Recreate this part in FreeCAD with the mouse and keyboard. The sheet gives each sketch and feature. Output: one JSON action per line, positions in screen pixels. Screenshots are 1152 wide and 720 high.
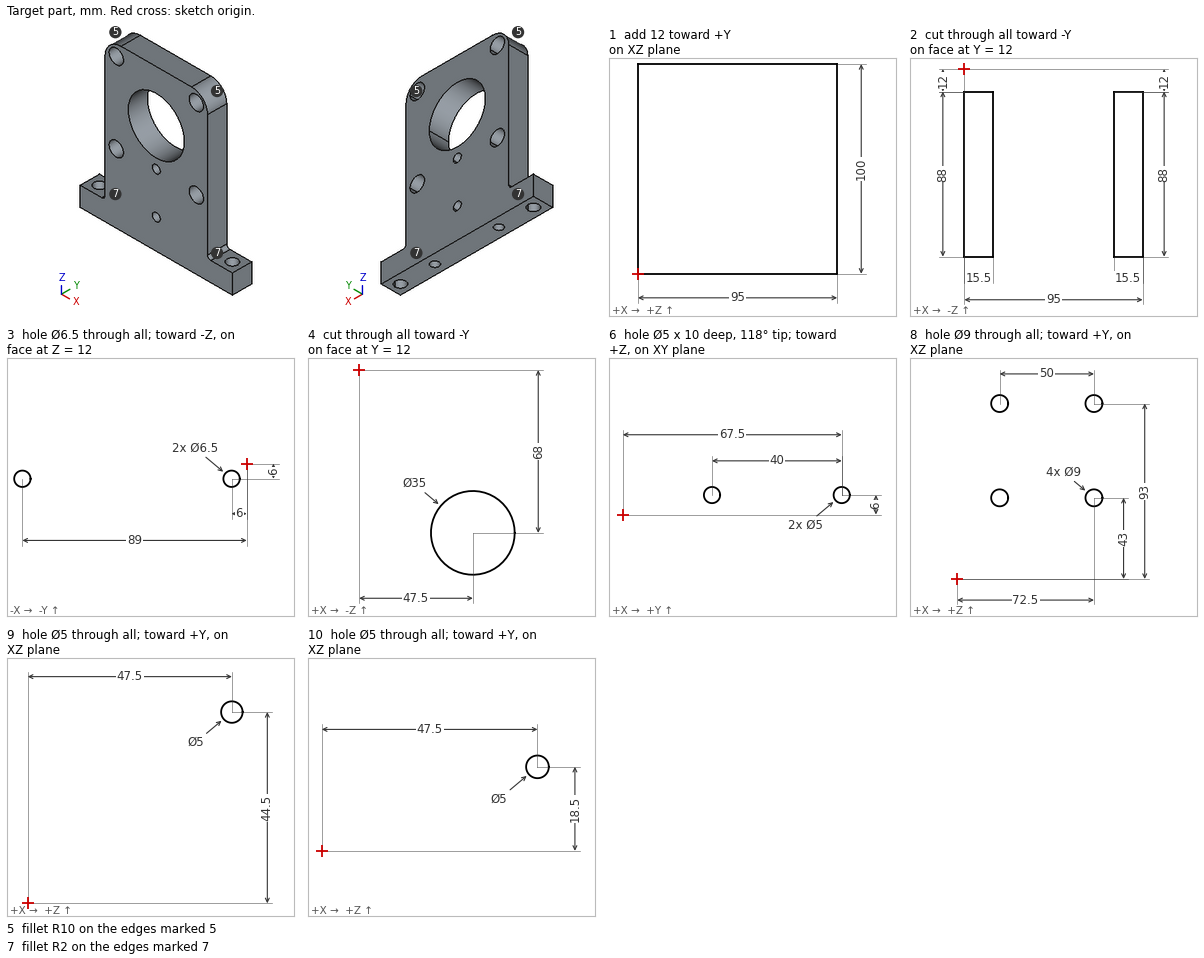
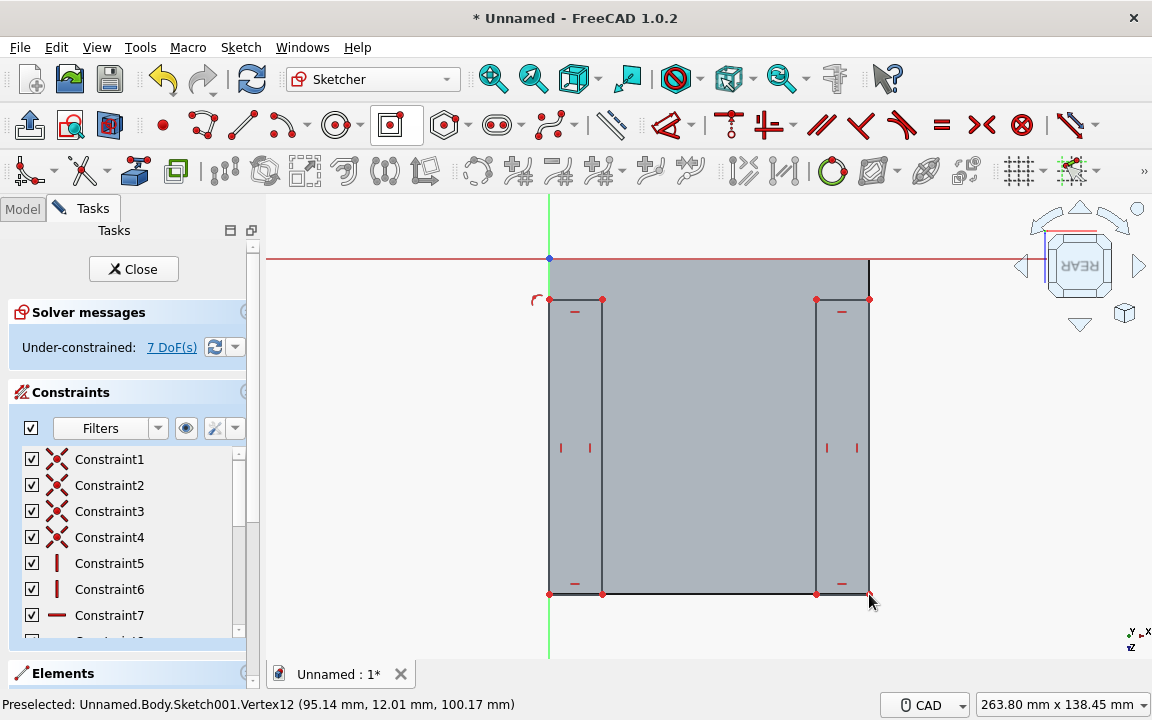
{"action": "left_click", "coordinate": [666, 126]}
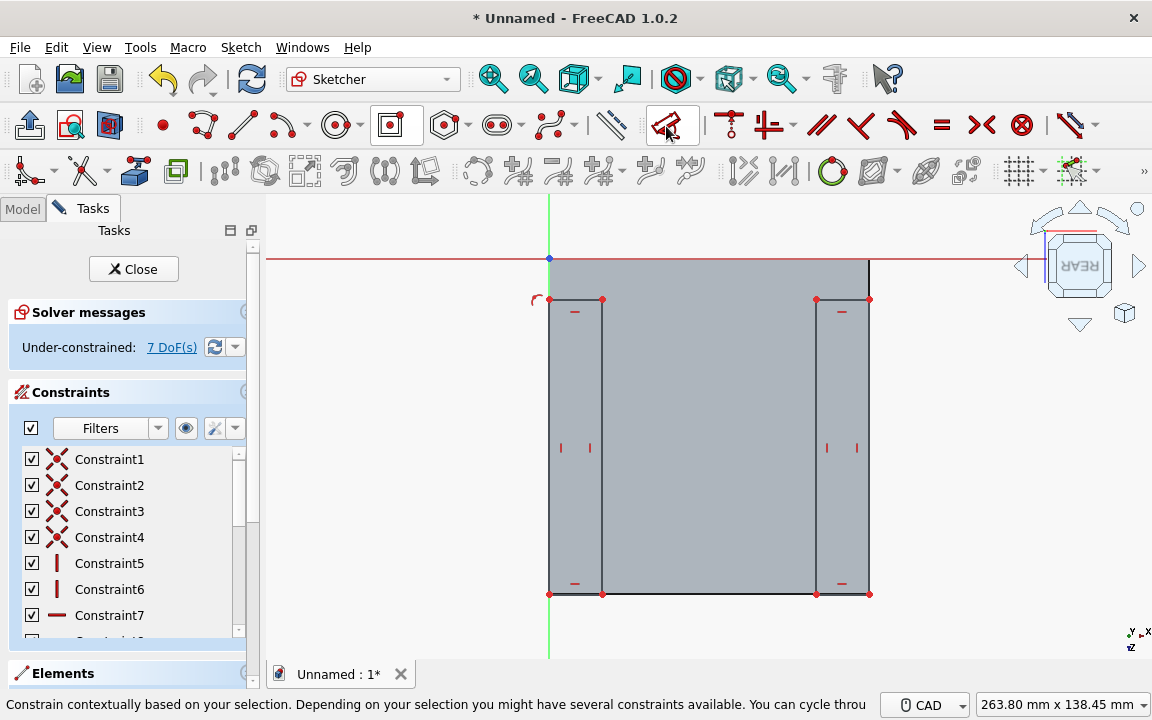
{"action": "left_click", "coordinate": [549, 389]}
{"action": "left_click", "coordinate": [515, 448]}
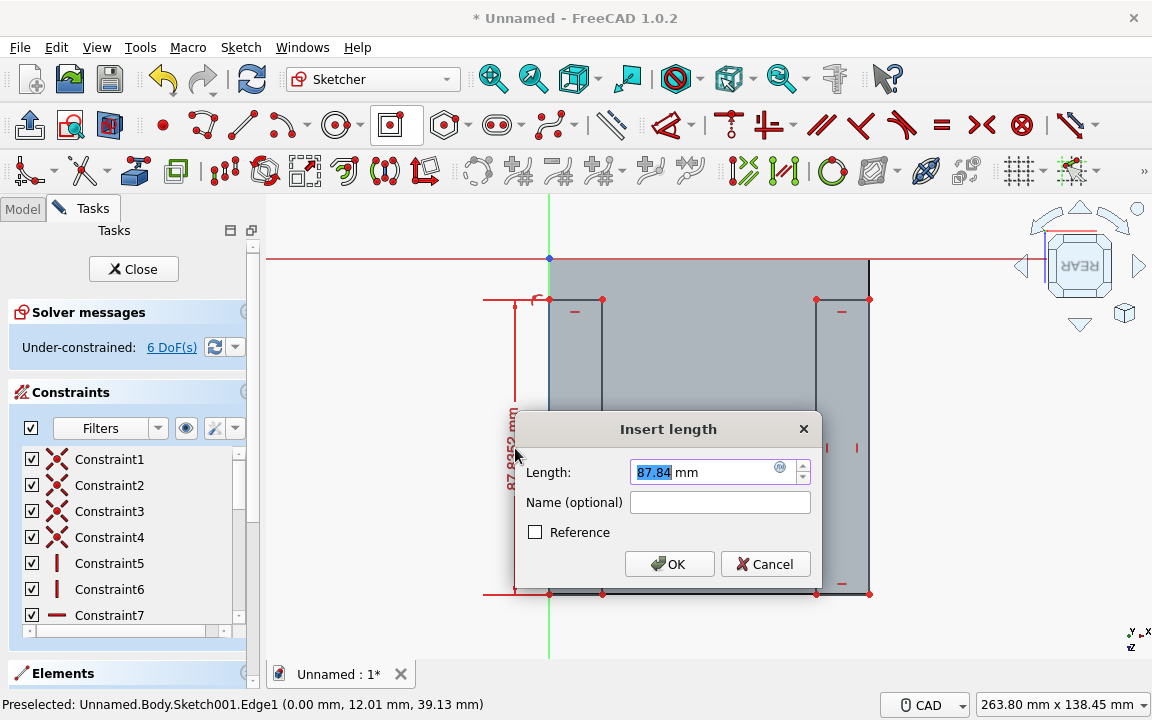
{"action": "type", "text": "88"}
{"action": "key", "text": "Return"}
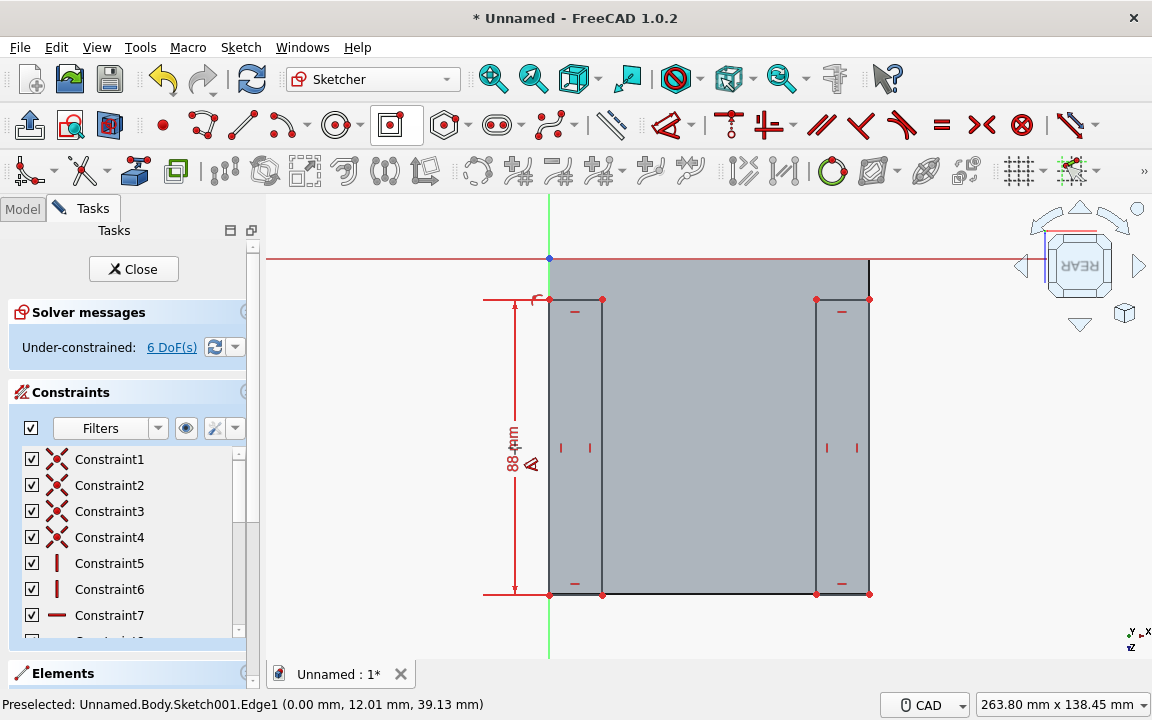
{"action": "left_click", "coordinate": [816, 389]}
{"action": "left_click", "coordinate": [850, 448]}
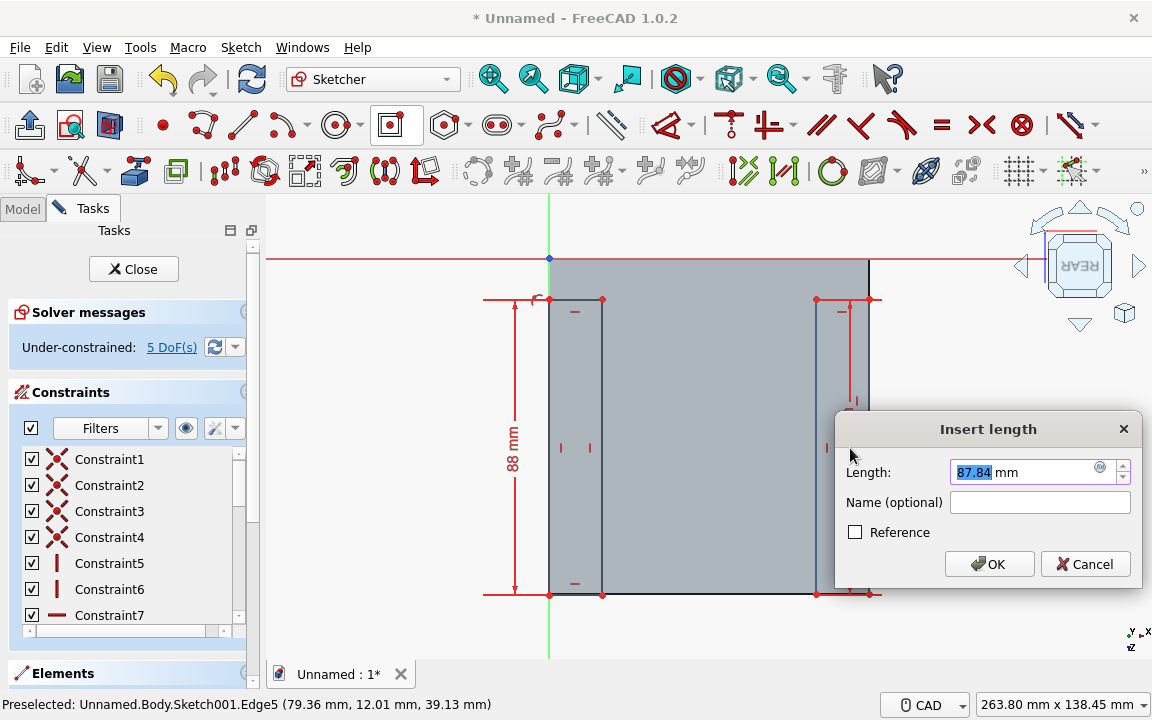
{"action": "type", "text": "88"}
{"action": "key", "text": "Return"}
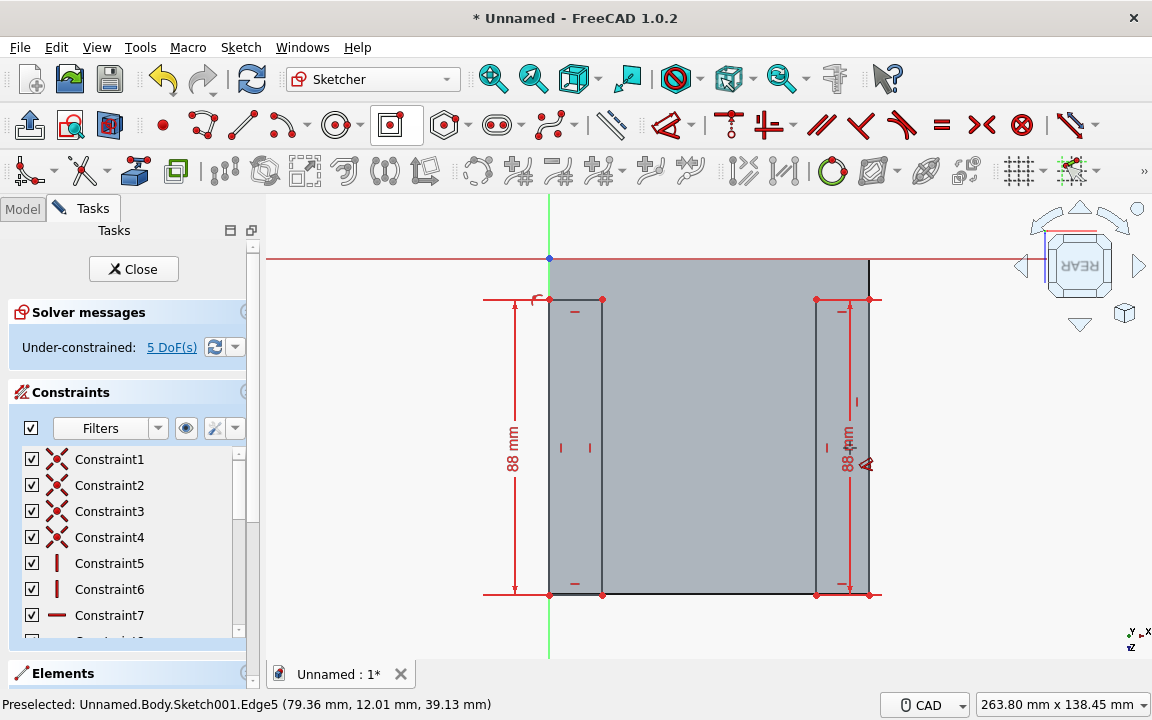
{"action": "left_click", "coordinate": [549, 300]}
{"action": "left_click", "coordinate": [515, 279]}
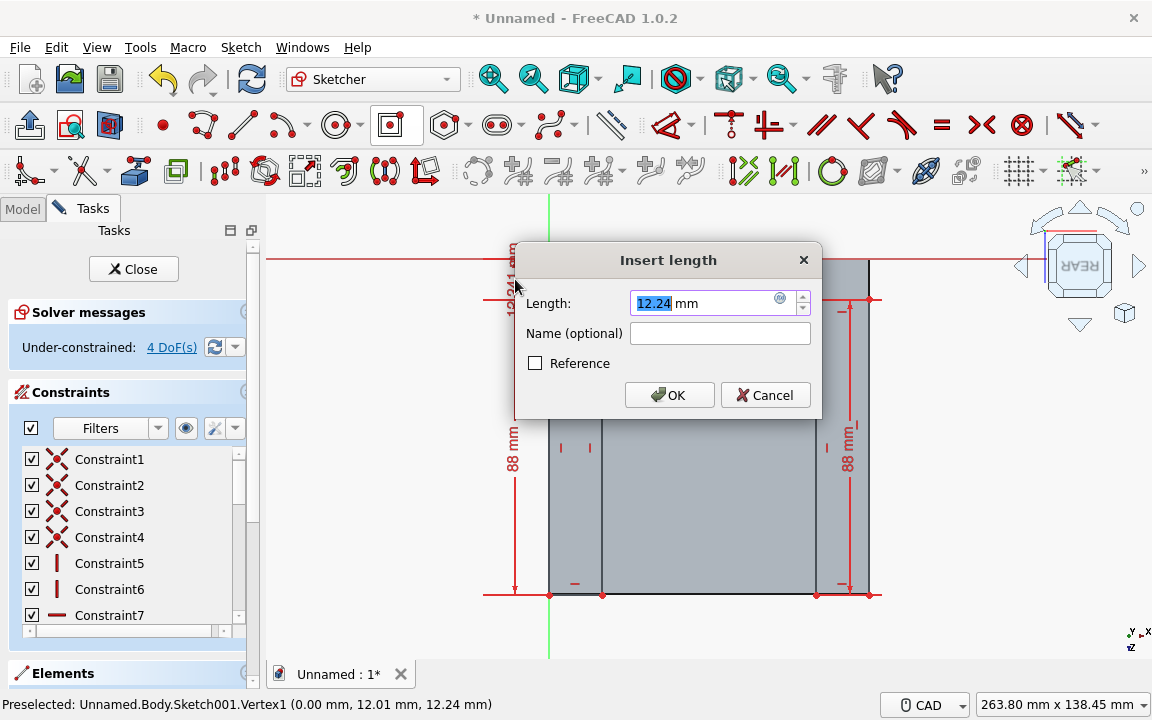
{"action": "type", "text": "12"}
{"action": "key", "text": "Return"}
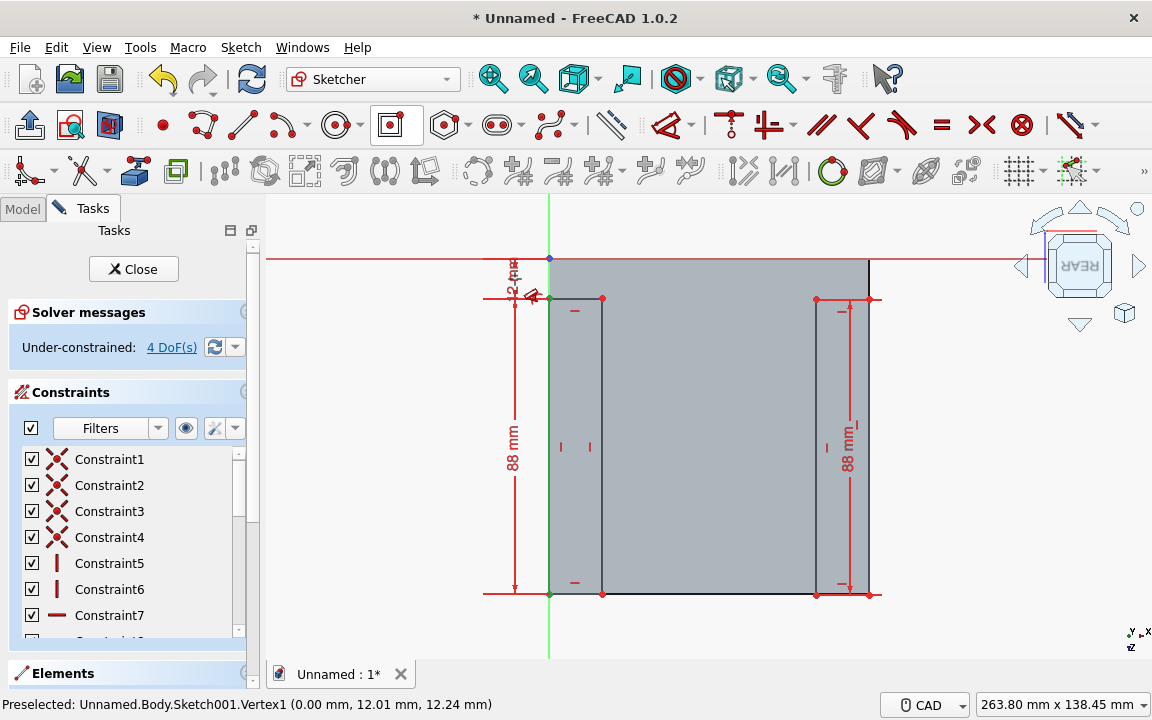
{"action": "left_click", "coordinate": [816, 300]}
{"action": "left_click", "coordinate": [850, 279]}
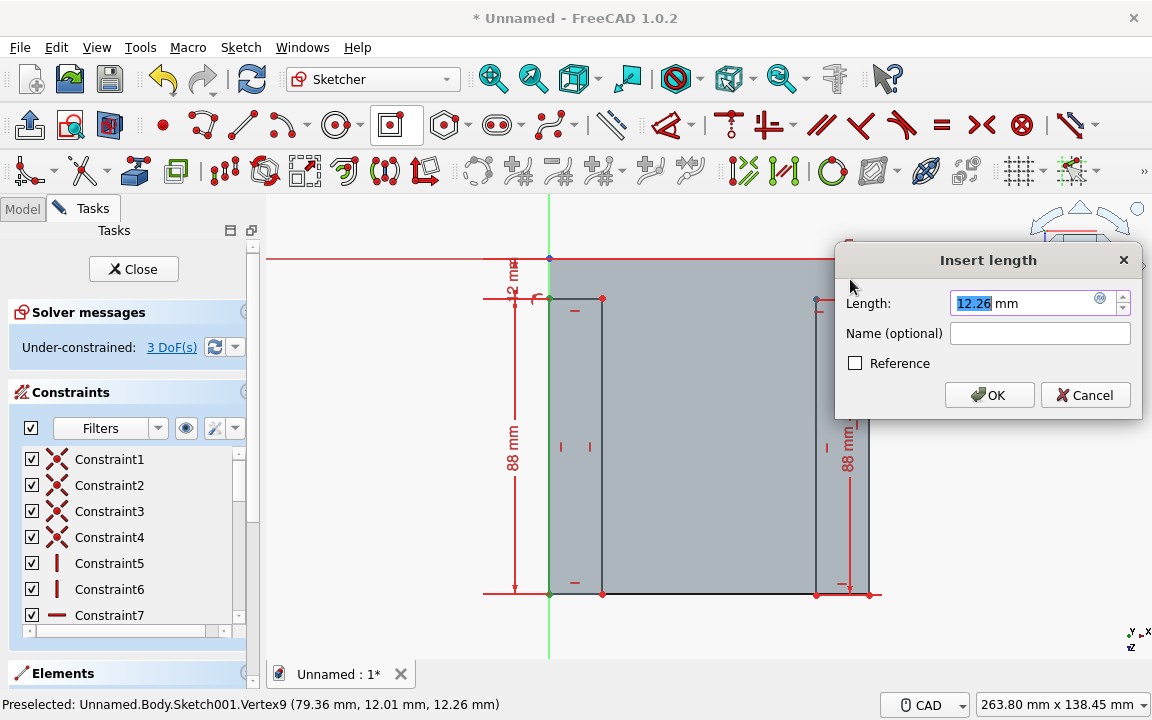
{"action": "type", "text": "12"}
{"action": "key", "text": "Return"}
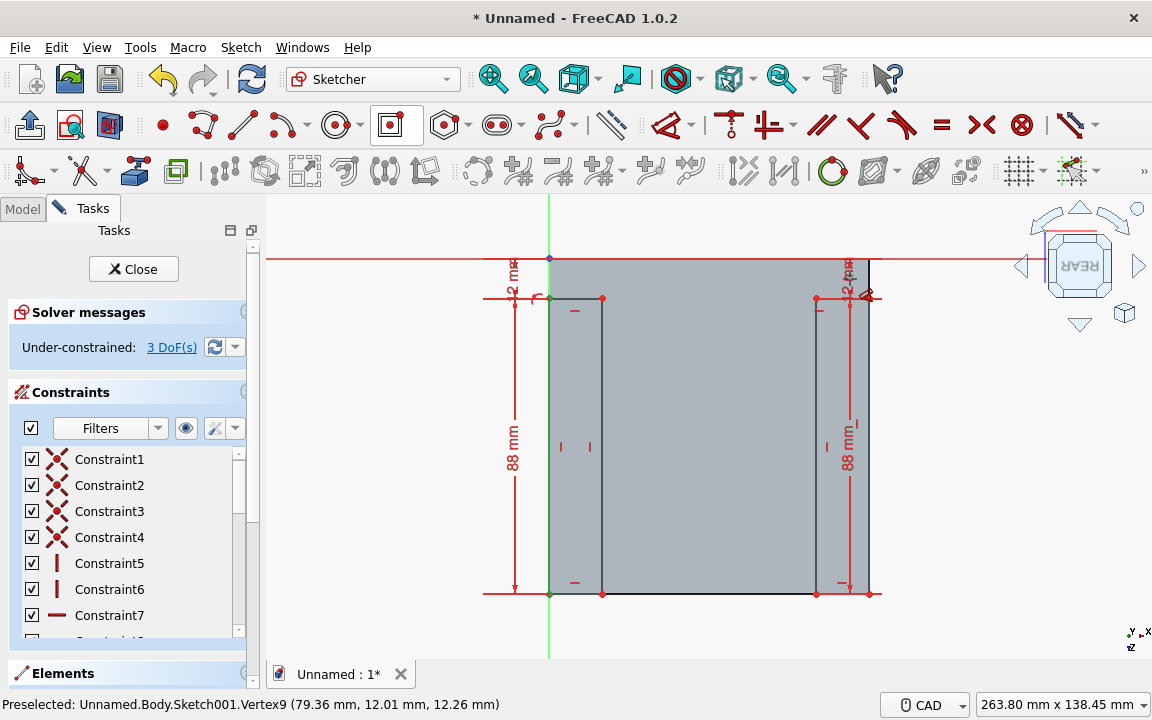
{"action": "left_click", "coordinate": [869, 594]}
{"action": "left_click", "coordinate": [709, 628]}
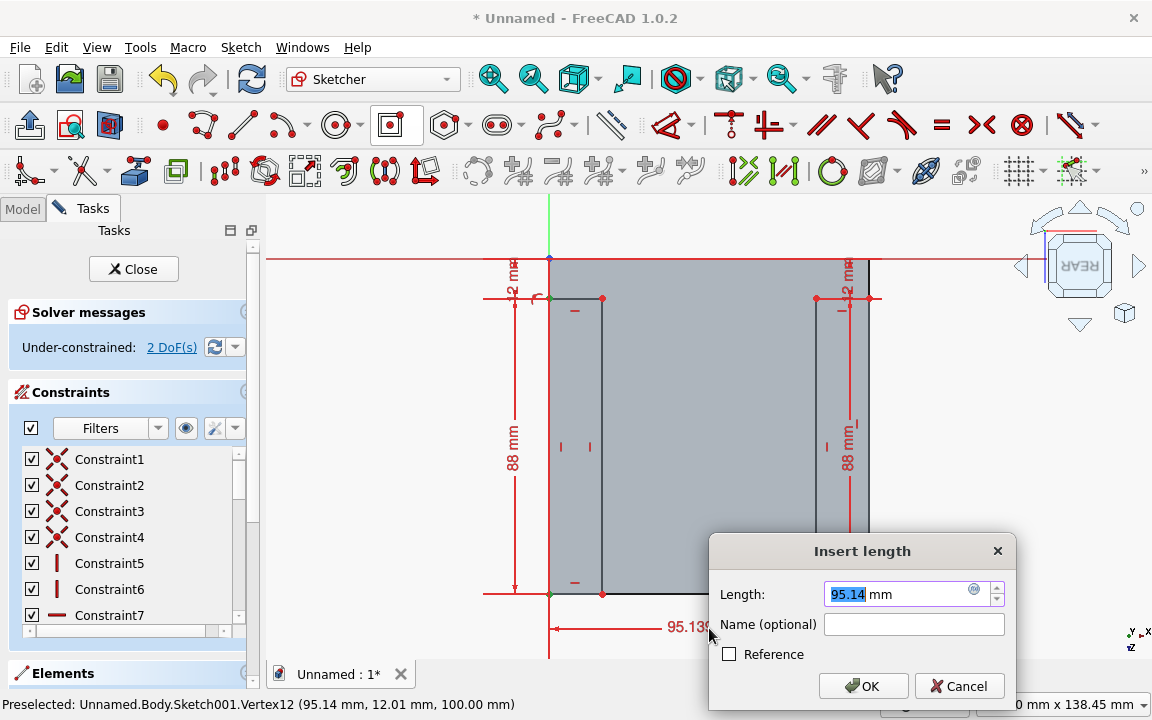
{"action": "type", "text": "95"}
{"action": "key", "text": "Return"}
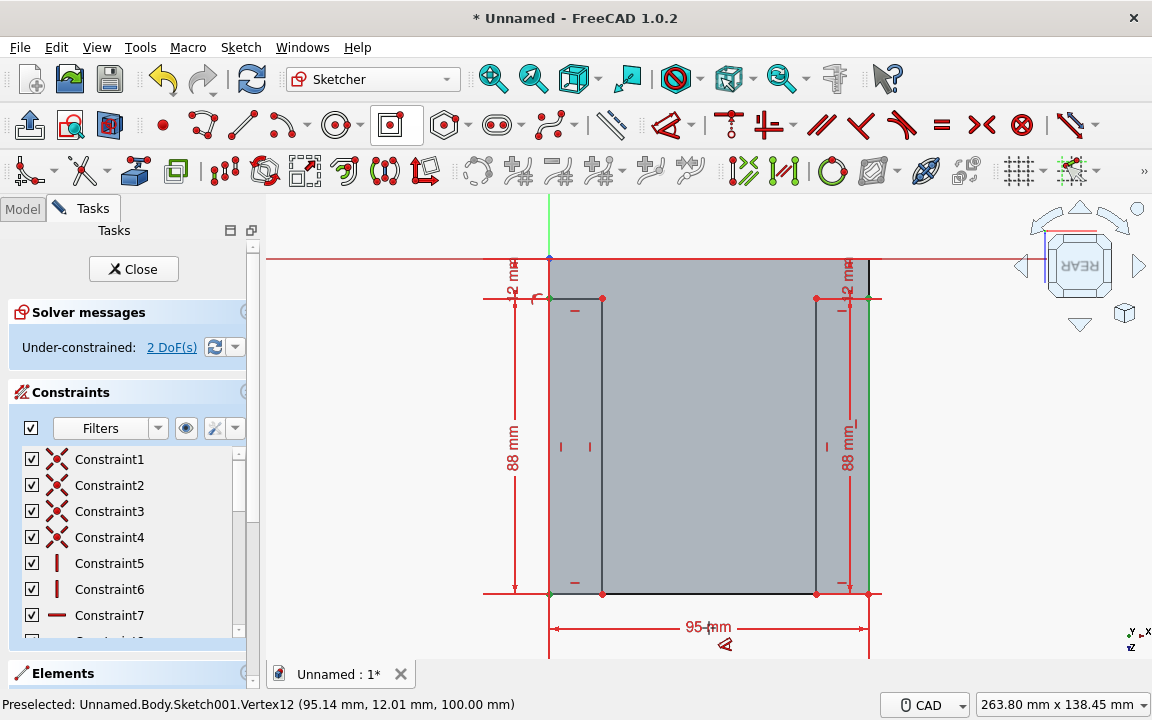
{"action": "left_click", "coordinate": [565, 594]}
{"action": "left_click", "coordinate": [576, 628]}